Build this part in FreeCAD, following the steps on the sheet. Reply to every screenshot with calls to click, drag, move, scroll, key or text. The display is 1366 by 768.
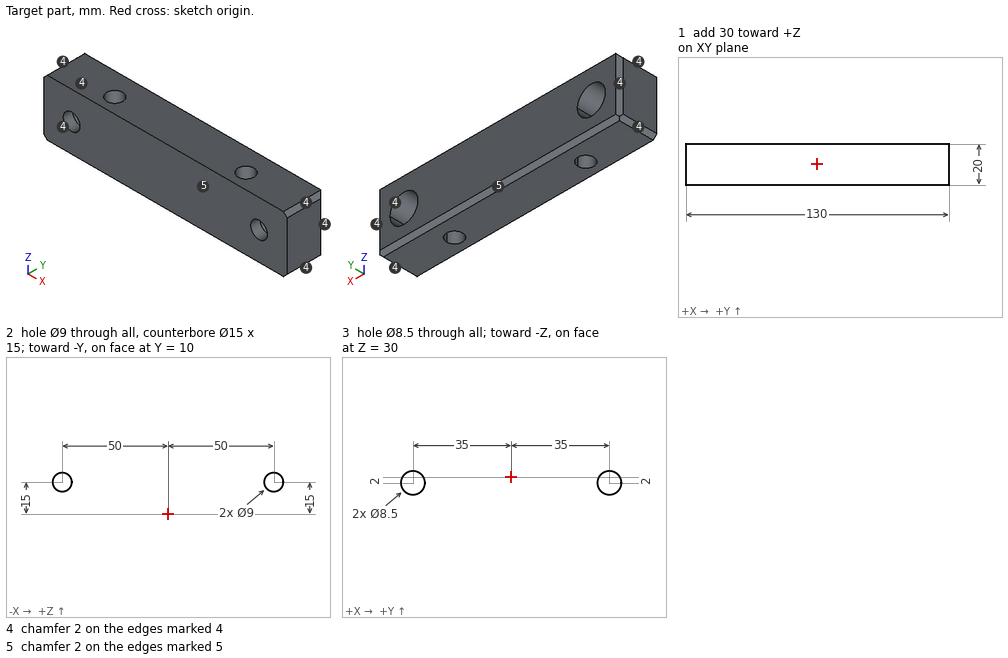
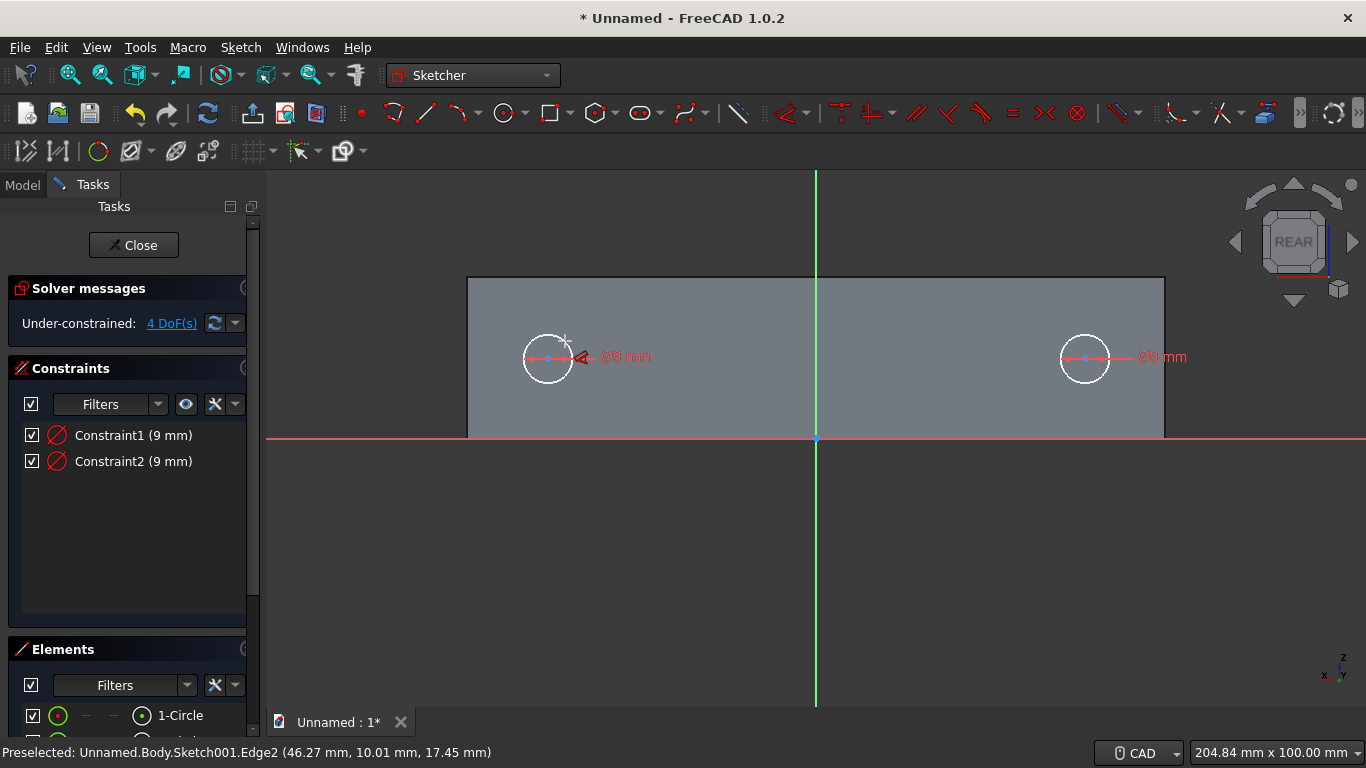
click(1085, 359)
click(950, 472)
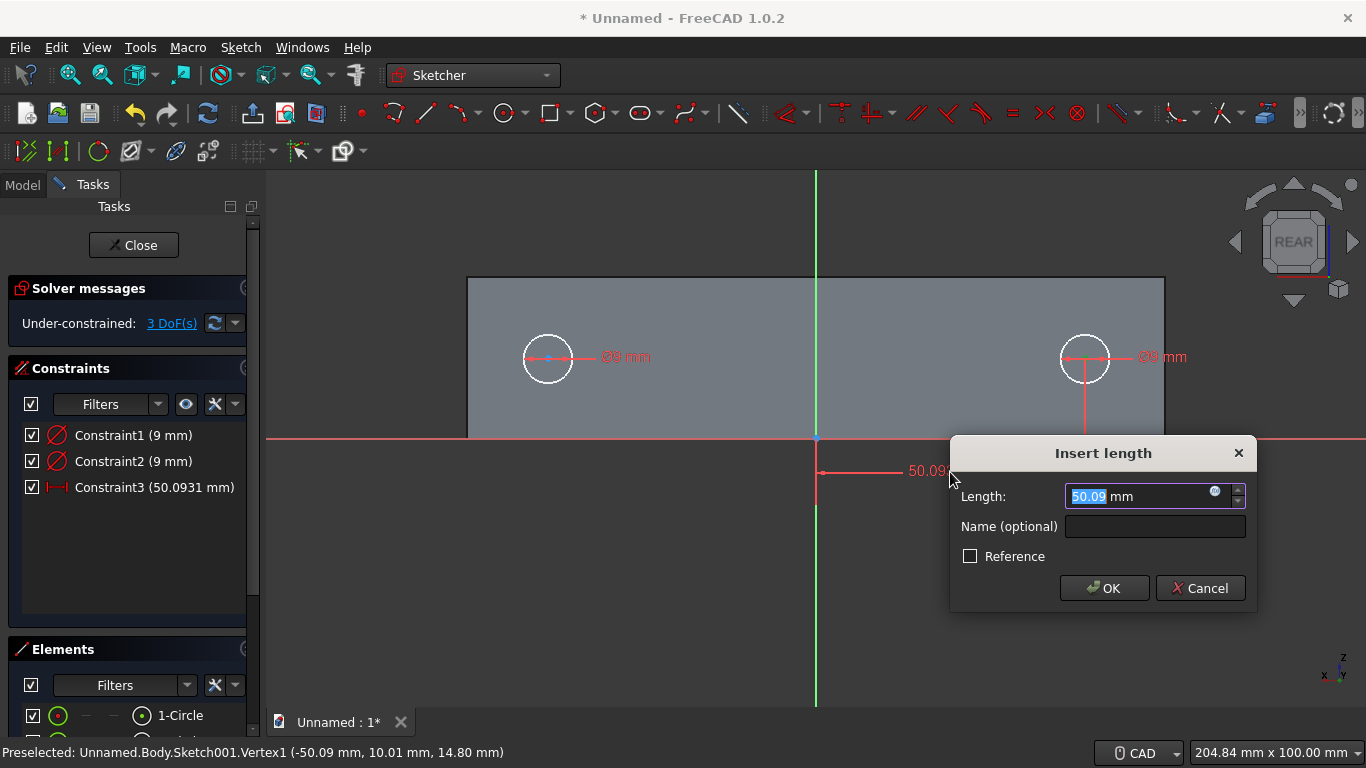
text(50)
key(Return)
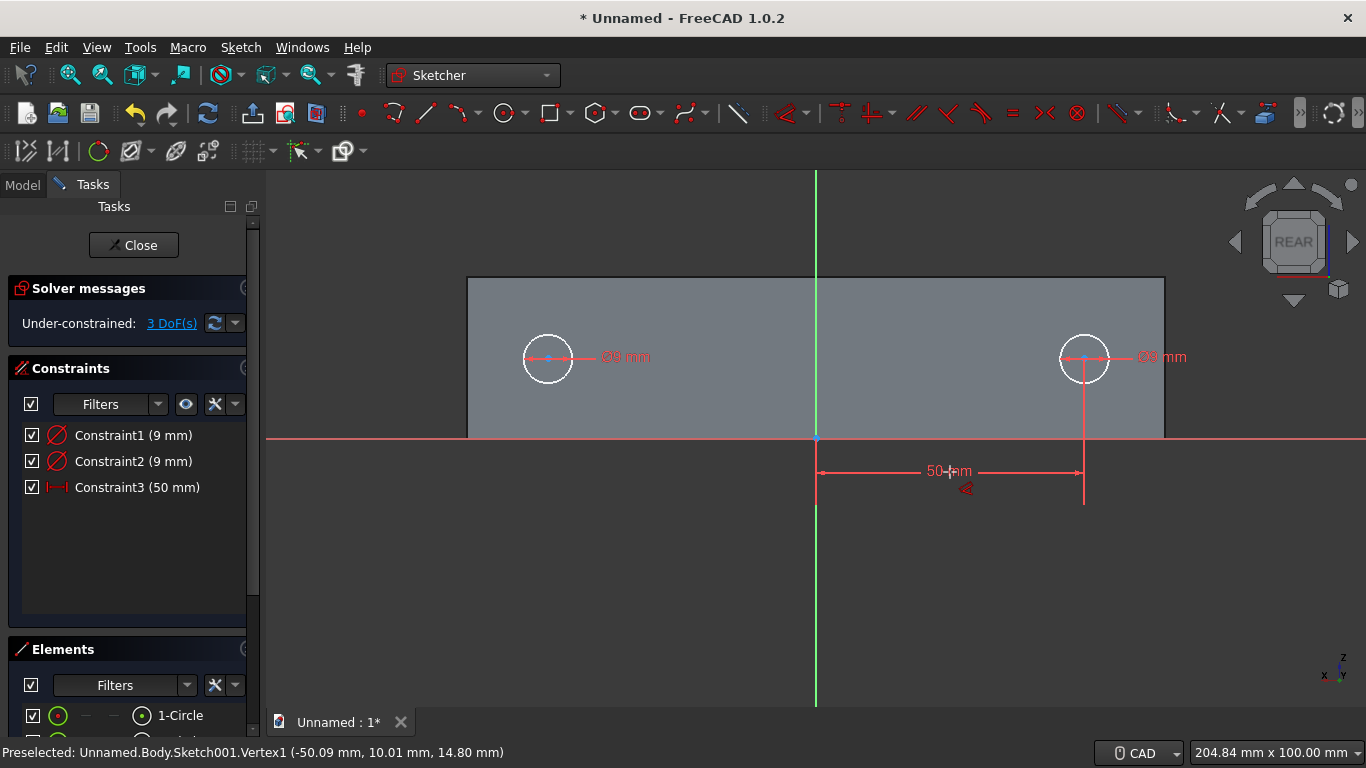
click(1085, 359)
click(1119, 399)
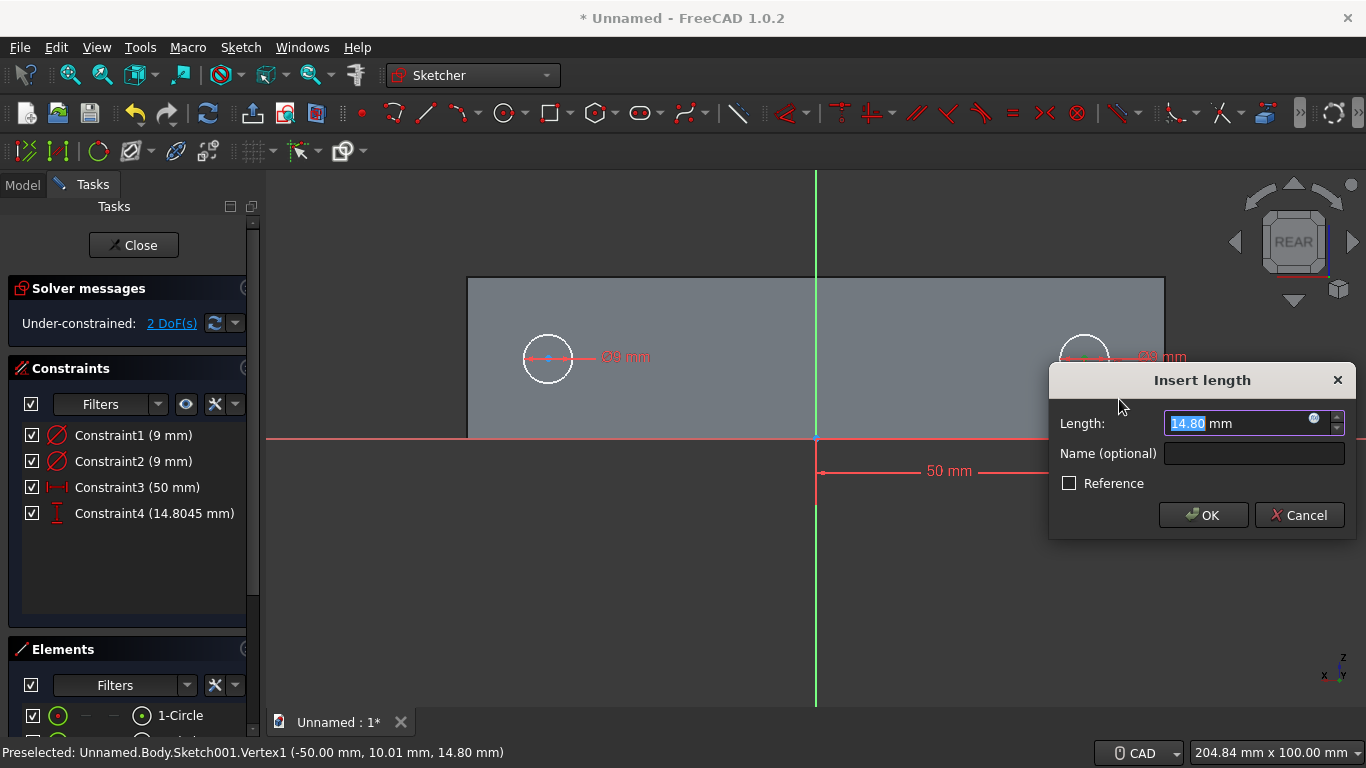
text(15)
key(Return)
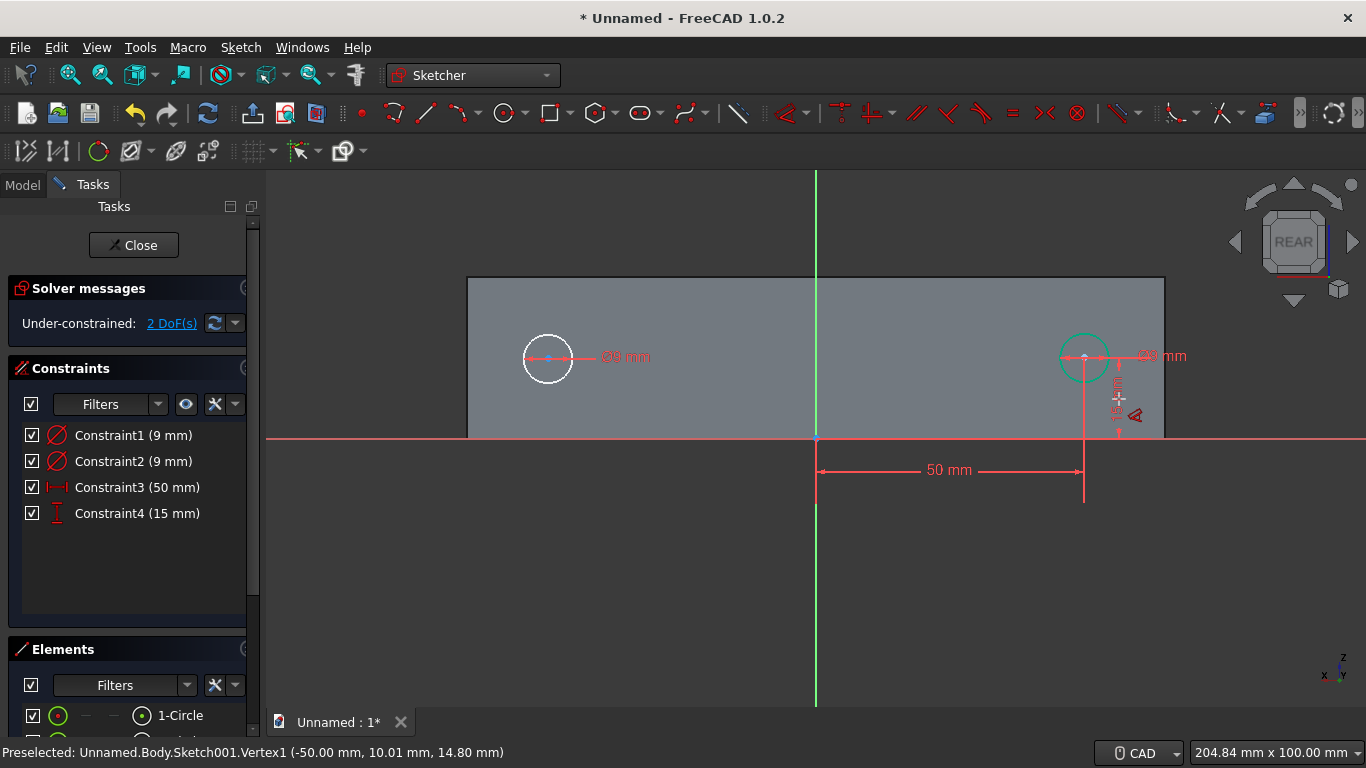
click(548, 359)
click(682, 472)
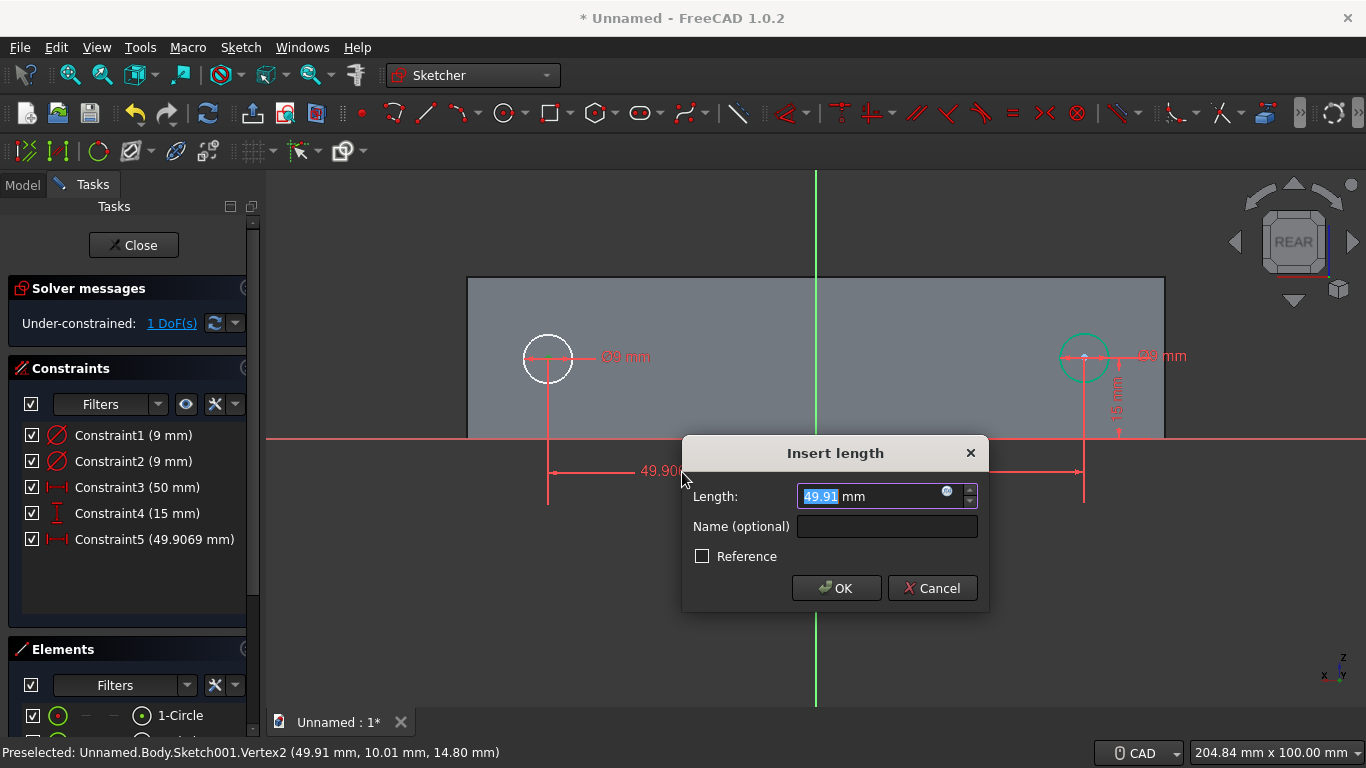
text(50)
key(Return)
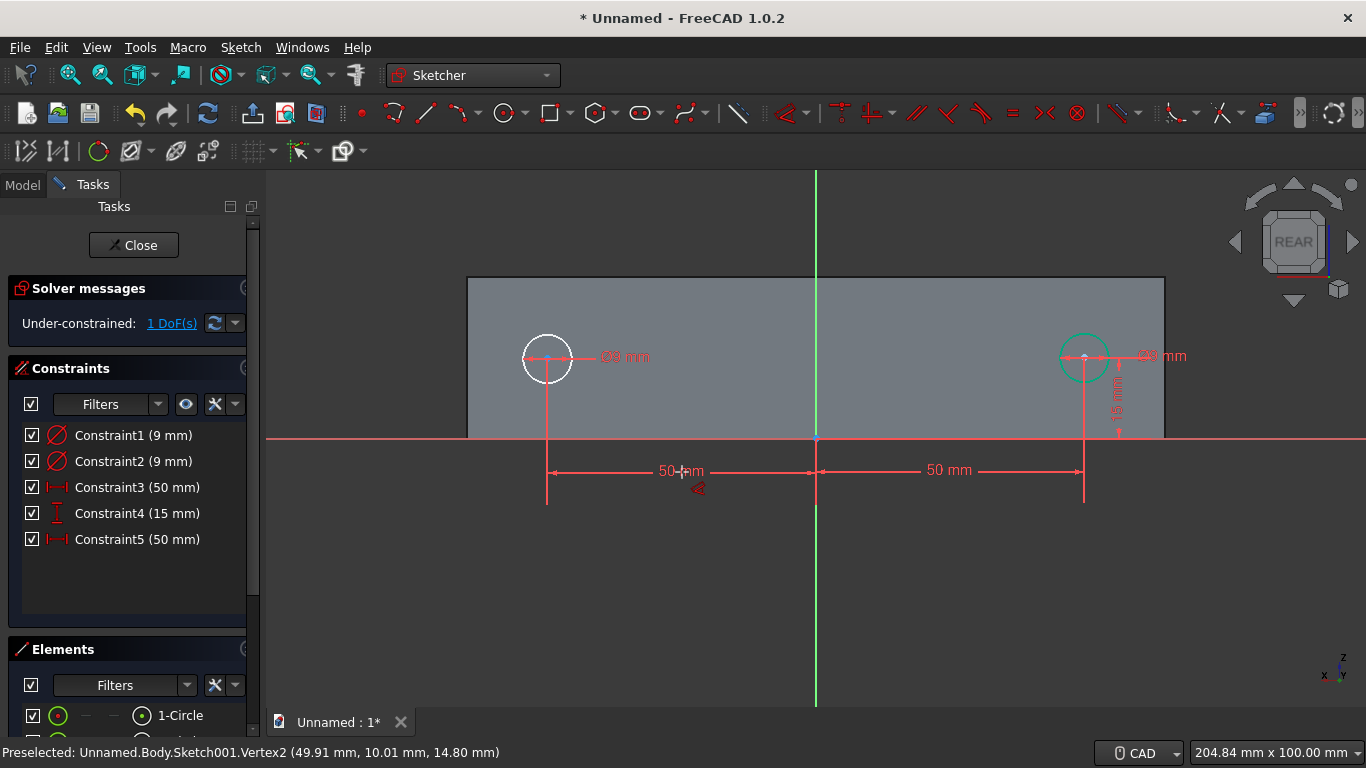
click(548, 359)
click(514, 399)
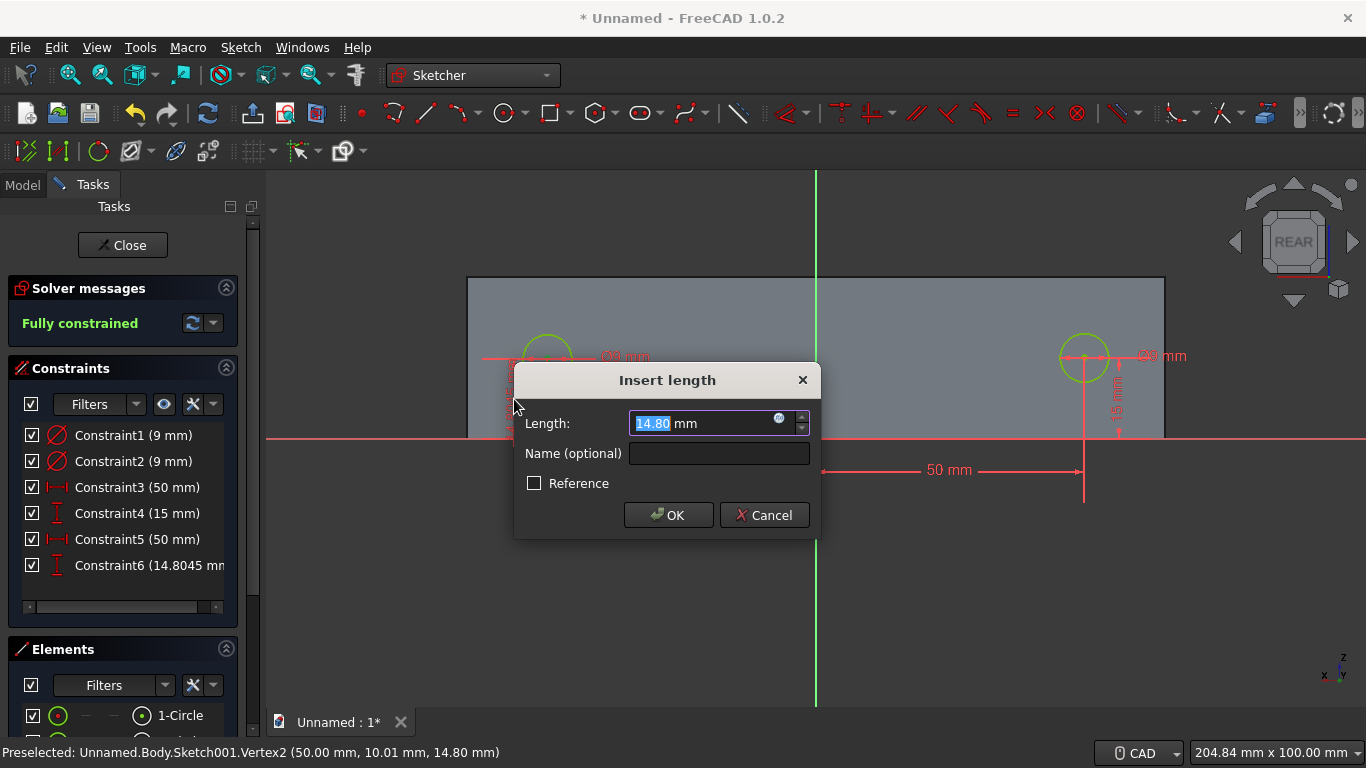
text(15)
key(Return)
key(Escape)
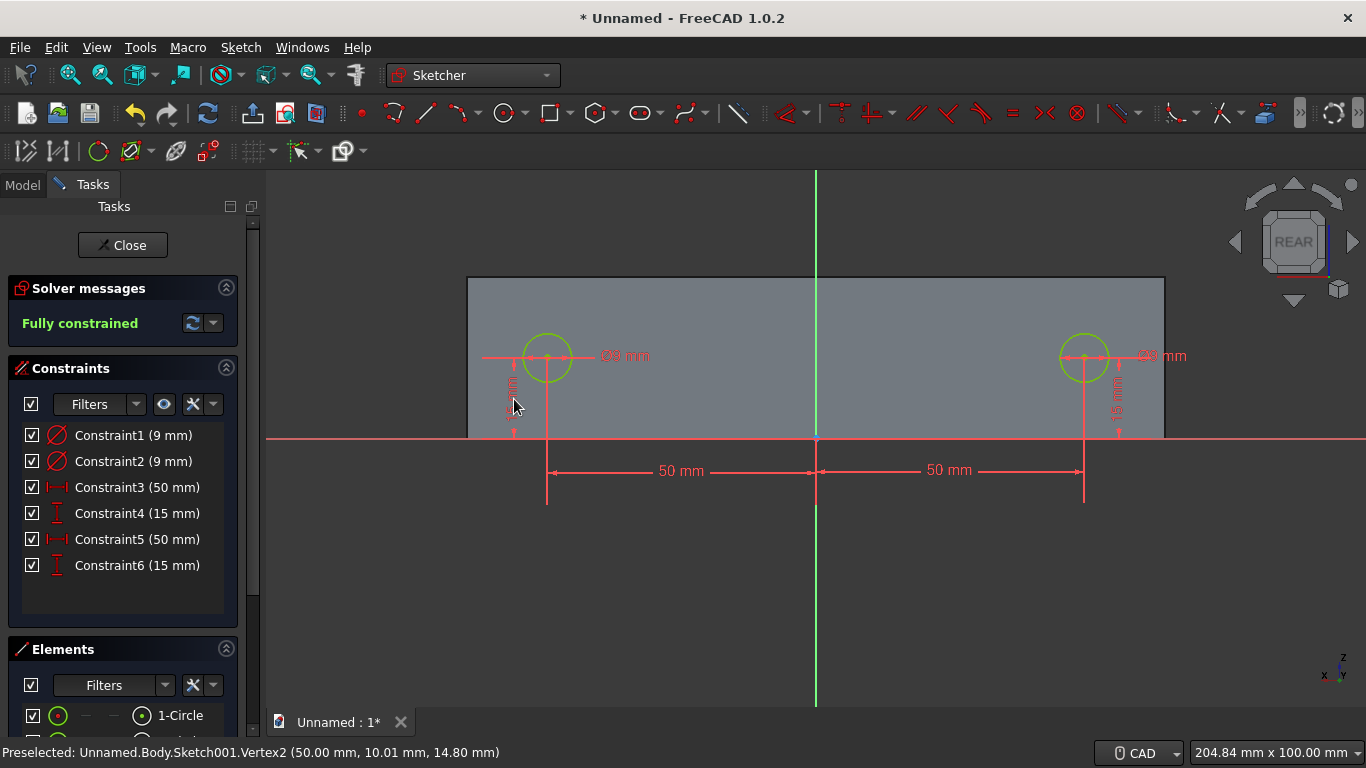
click(123, 245)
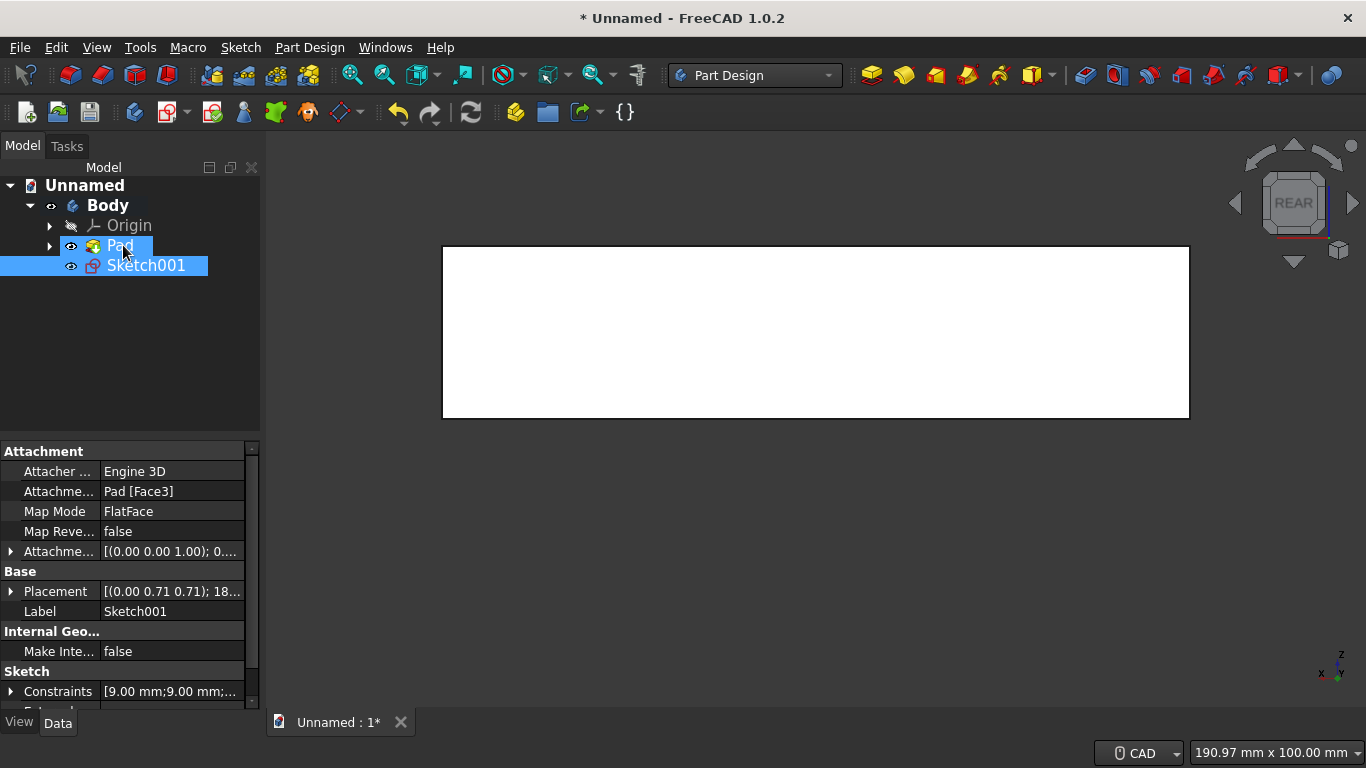
click(1118, 76)